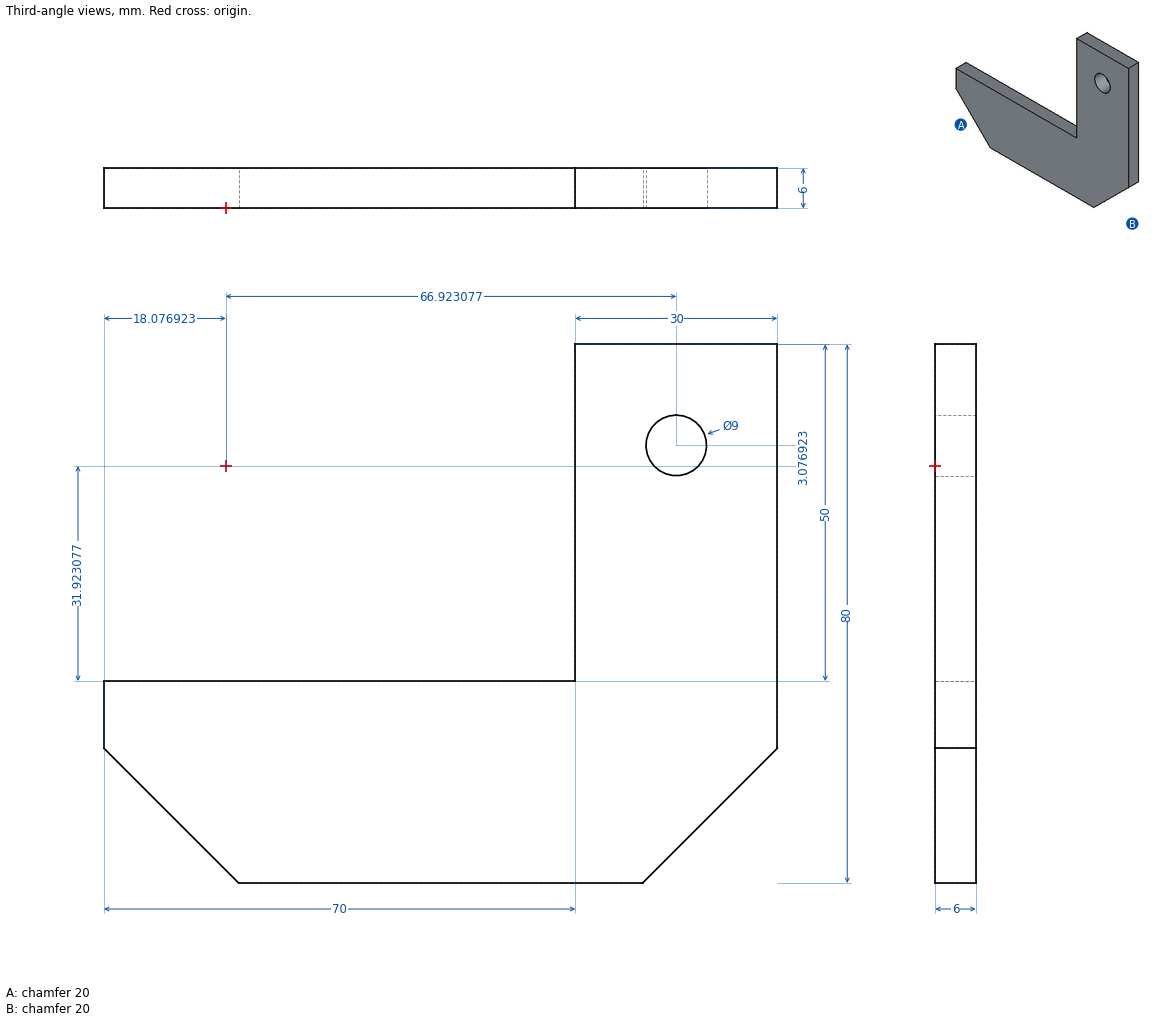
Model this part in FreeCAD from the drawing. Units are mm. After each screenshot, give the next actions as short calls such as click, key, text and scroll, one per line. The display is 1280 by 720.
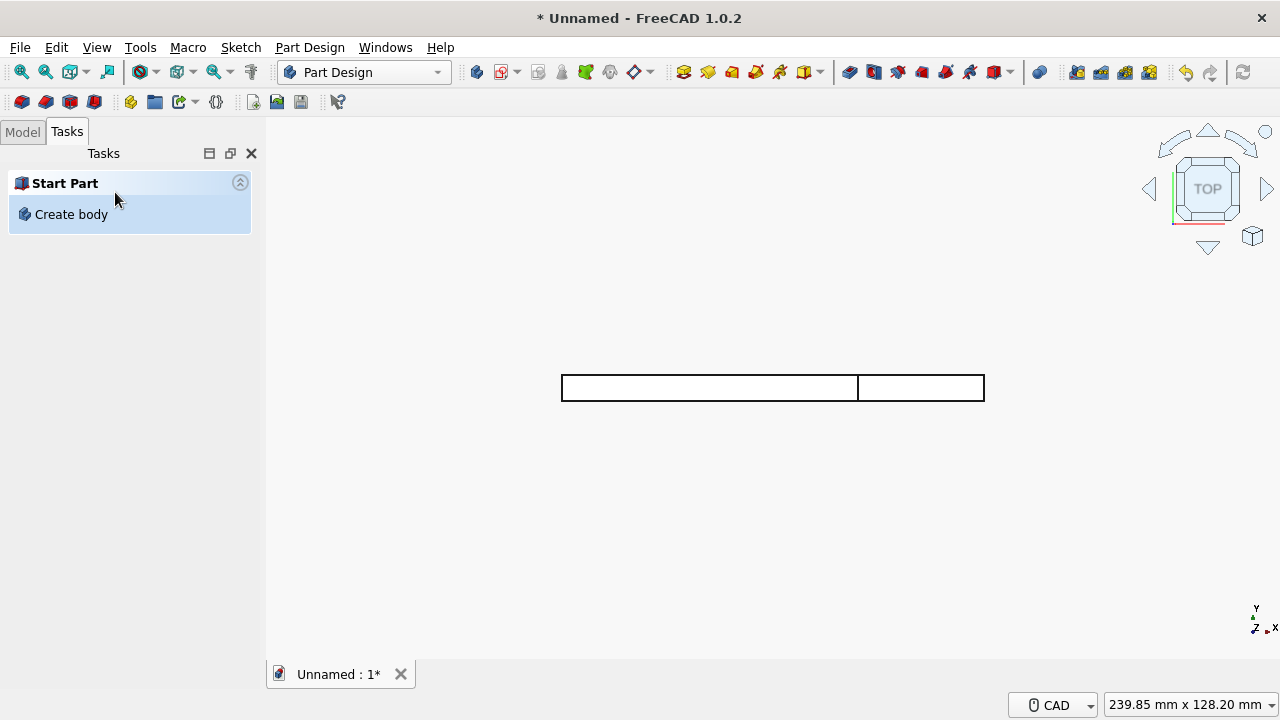
click(22, 72)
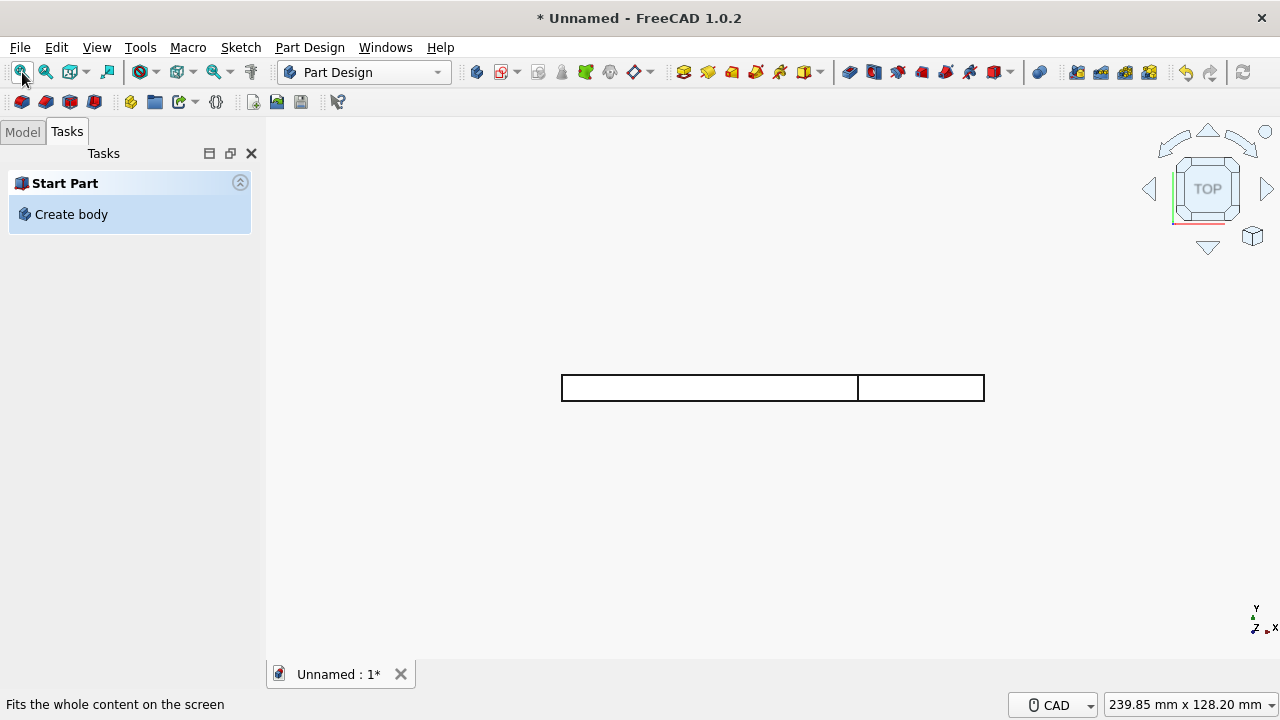
key(1)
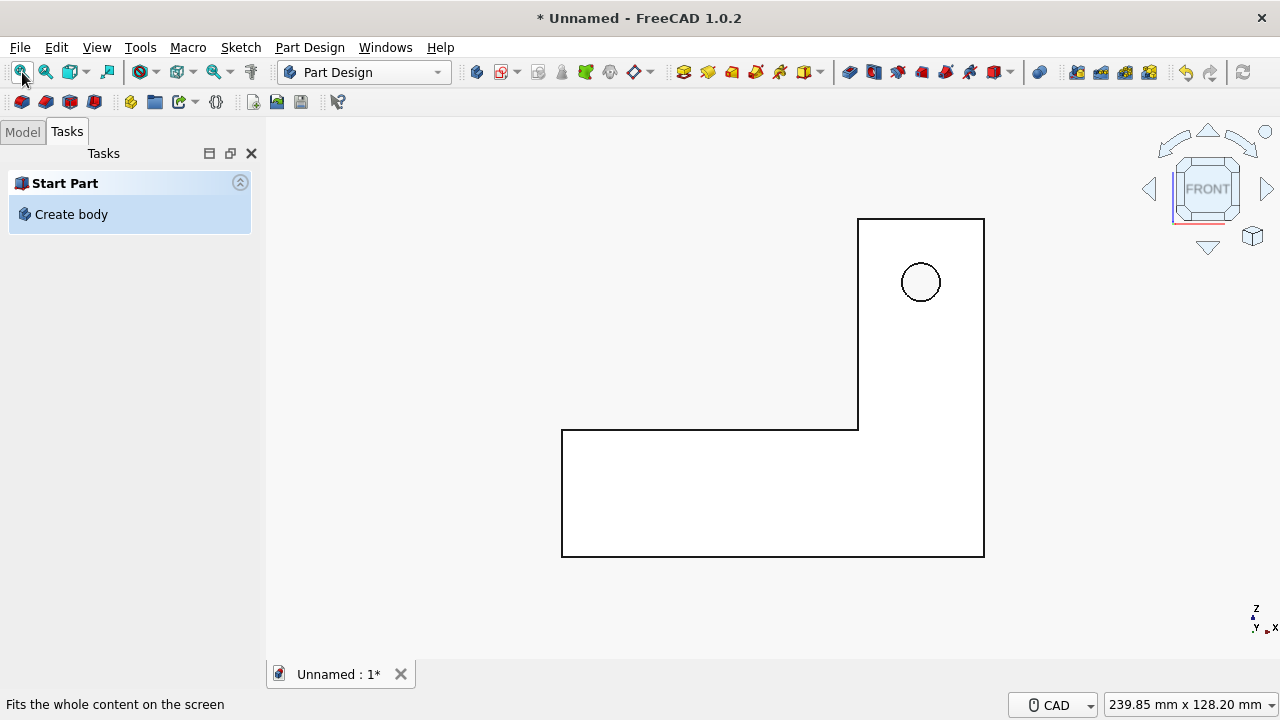
key(3)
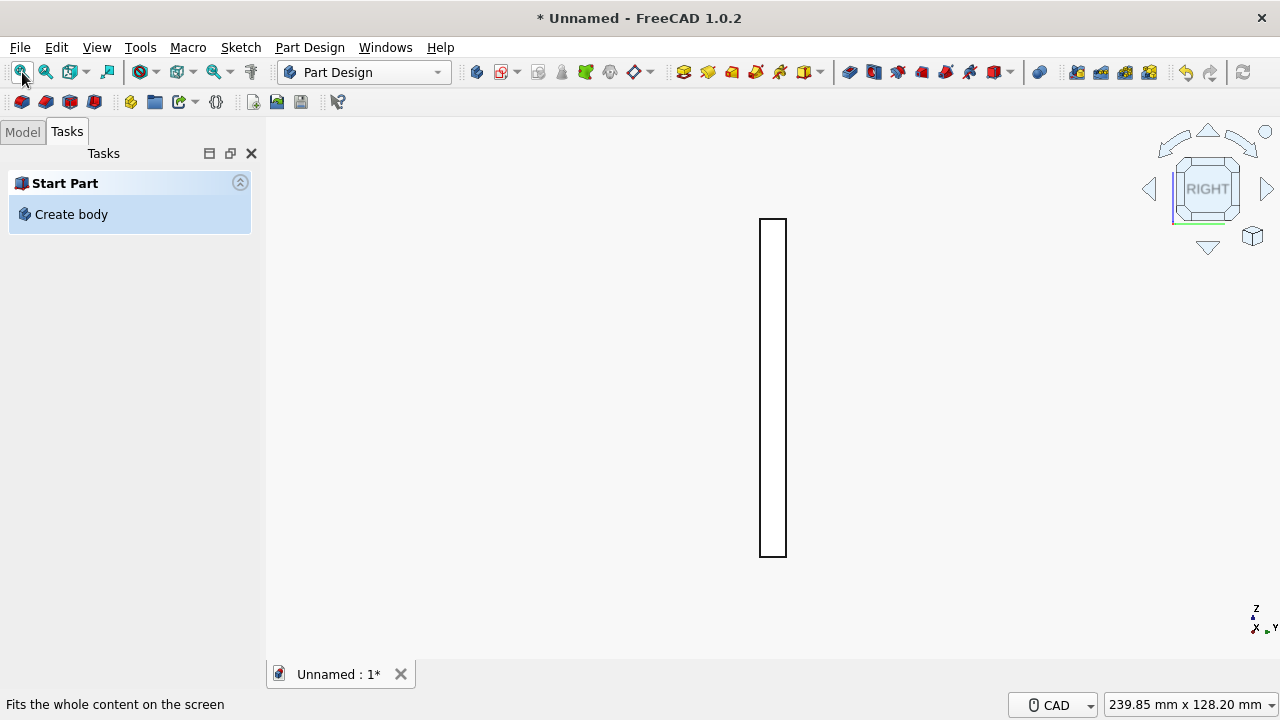
key(5)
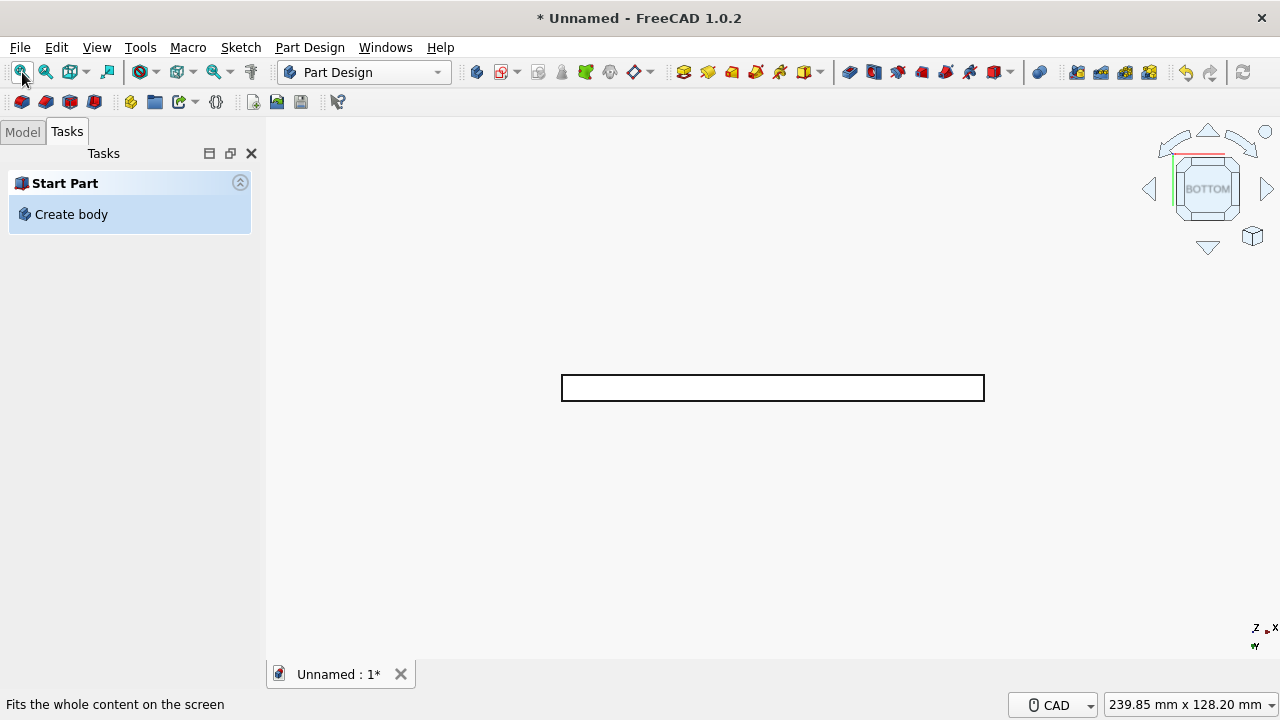
click(22, 72)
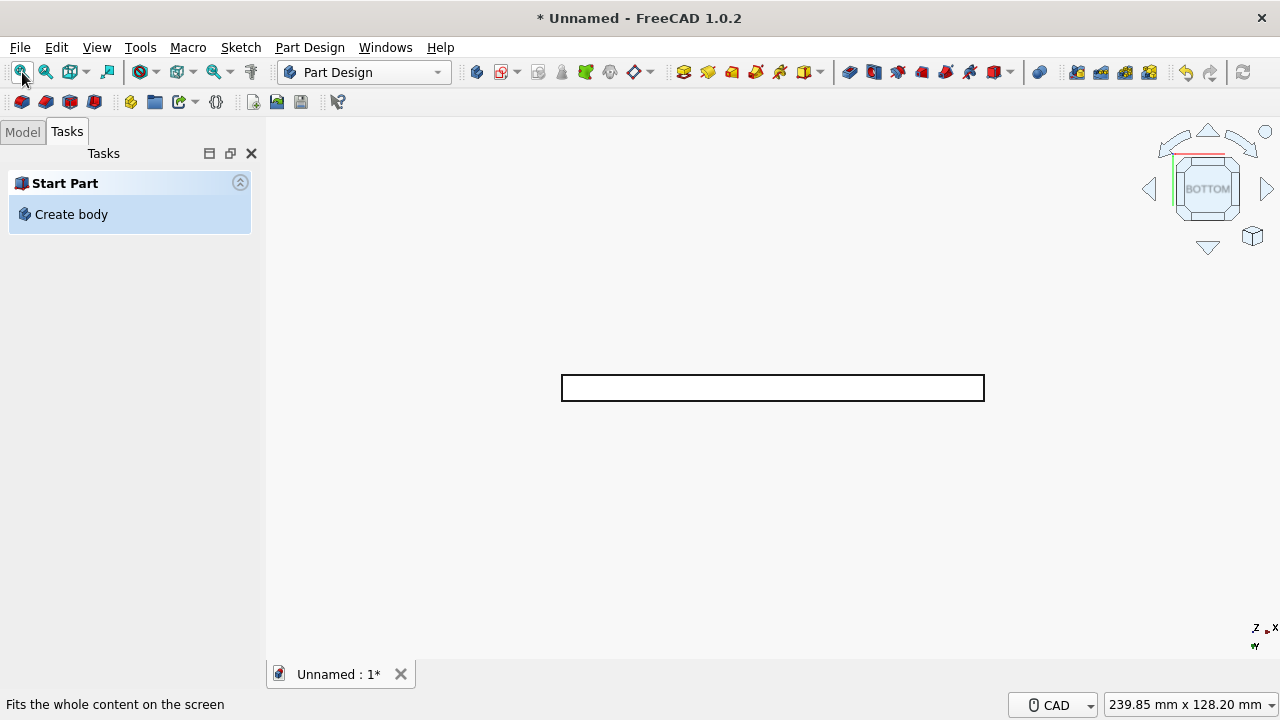
click(562, 387)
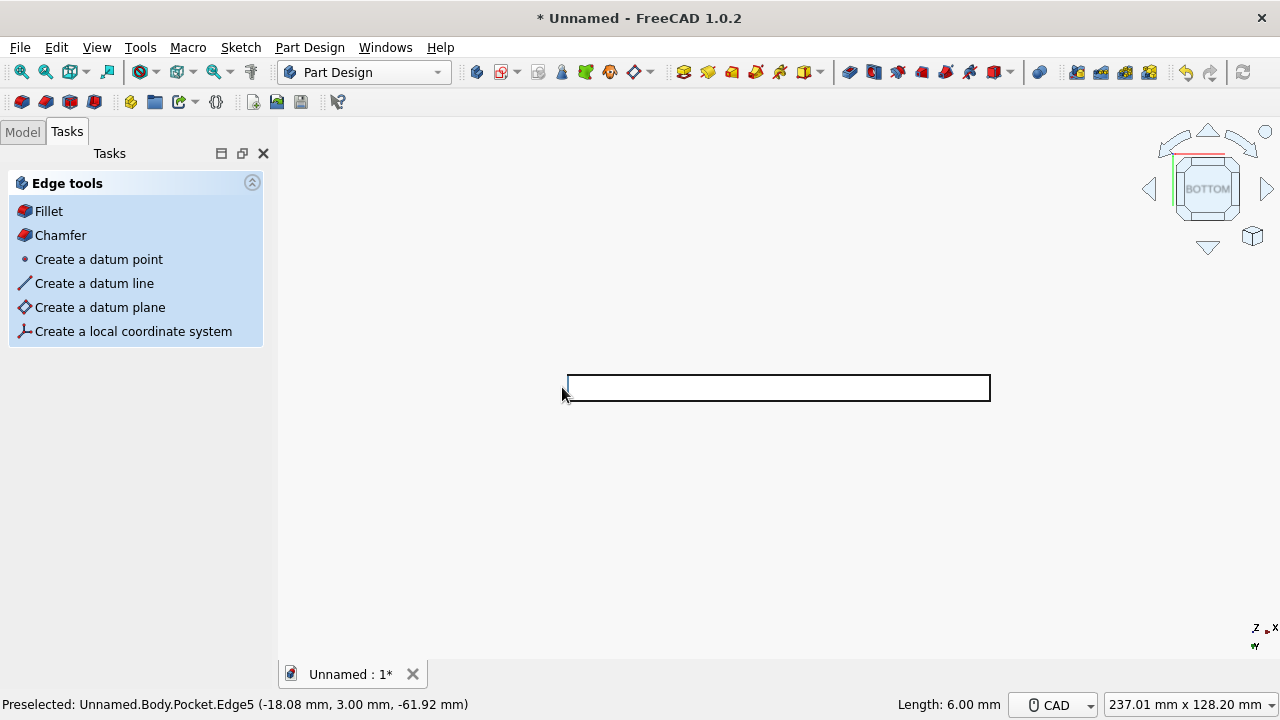
click(46, 102)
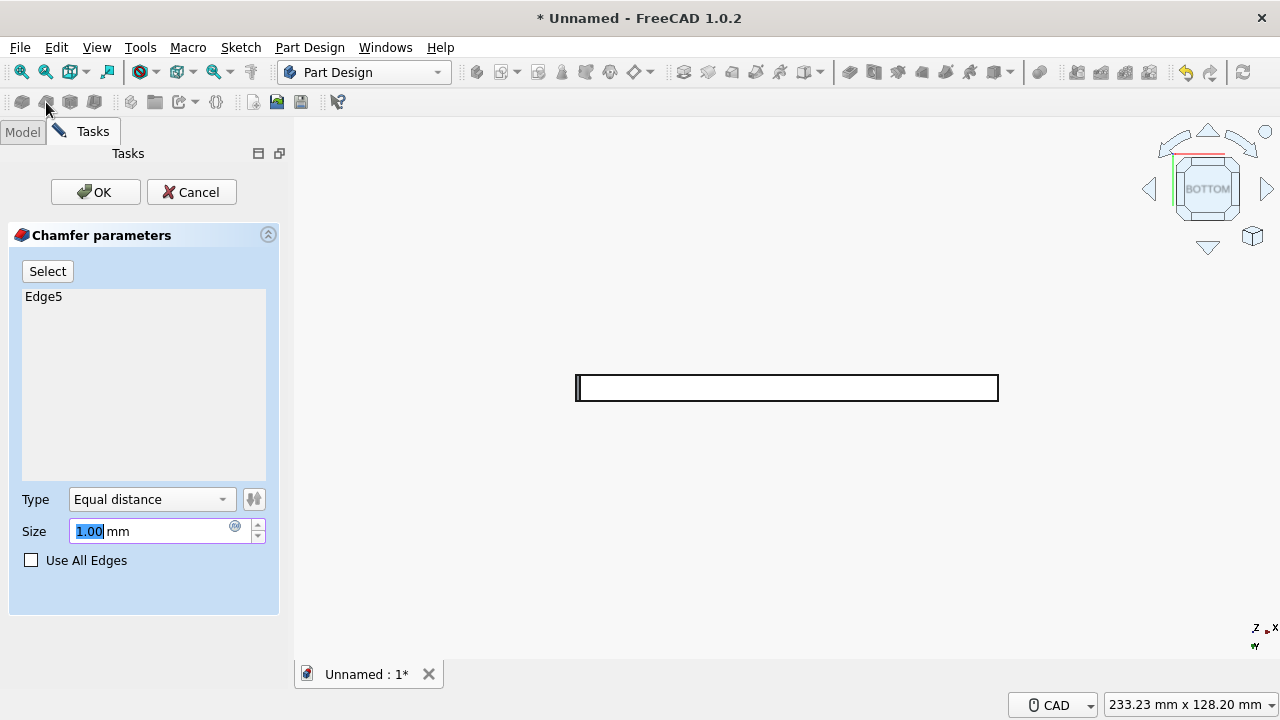
text(20)
key(Tab)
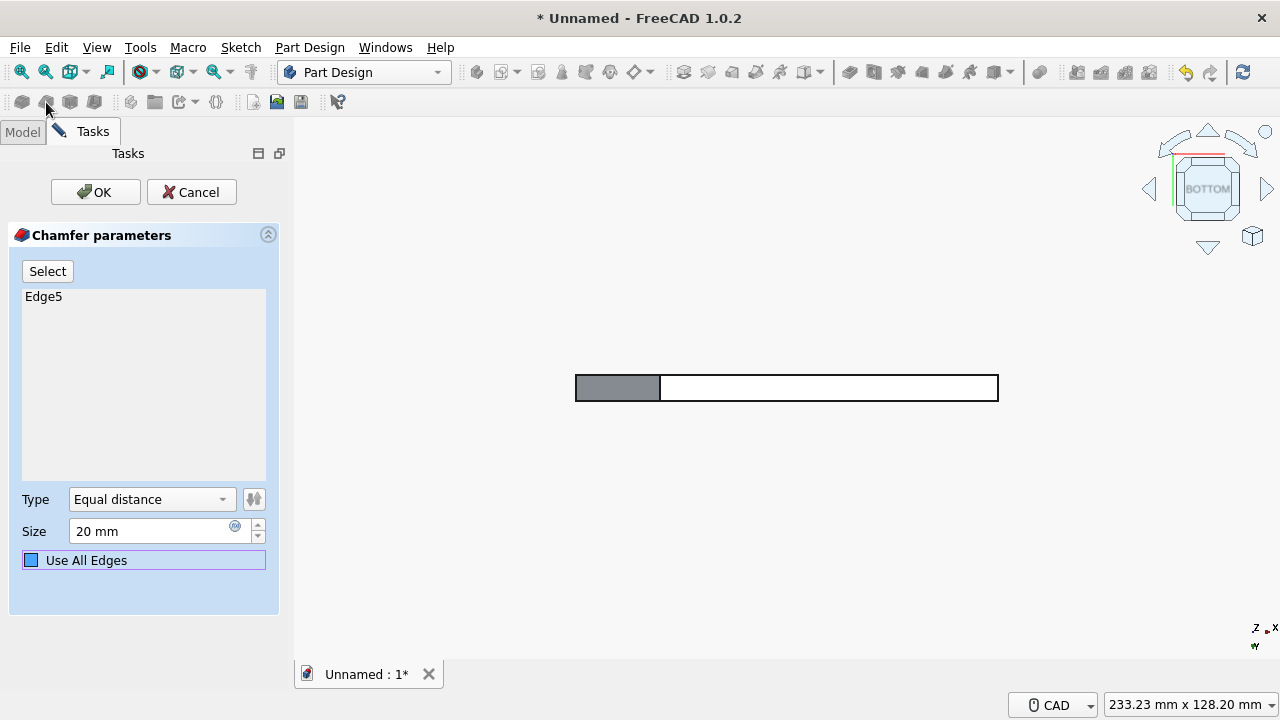
click(96, 192)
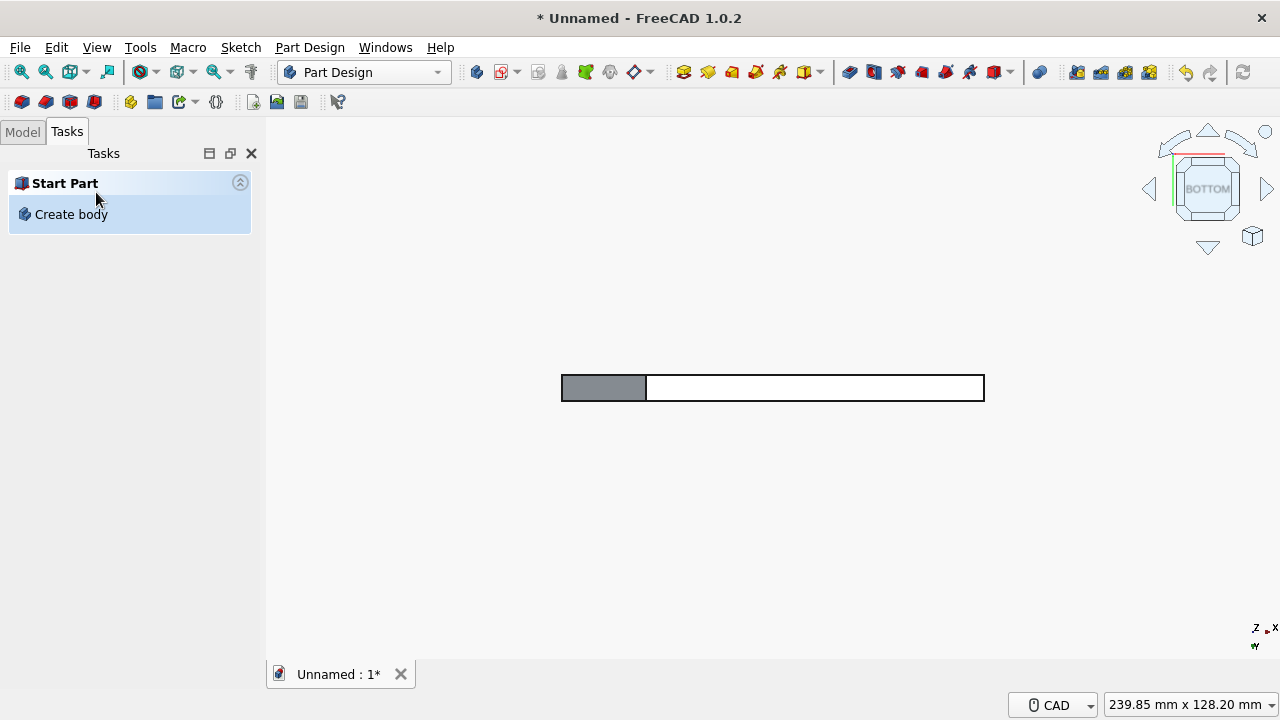
key(v)
key(f)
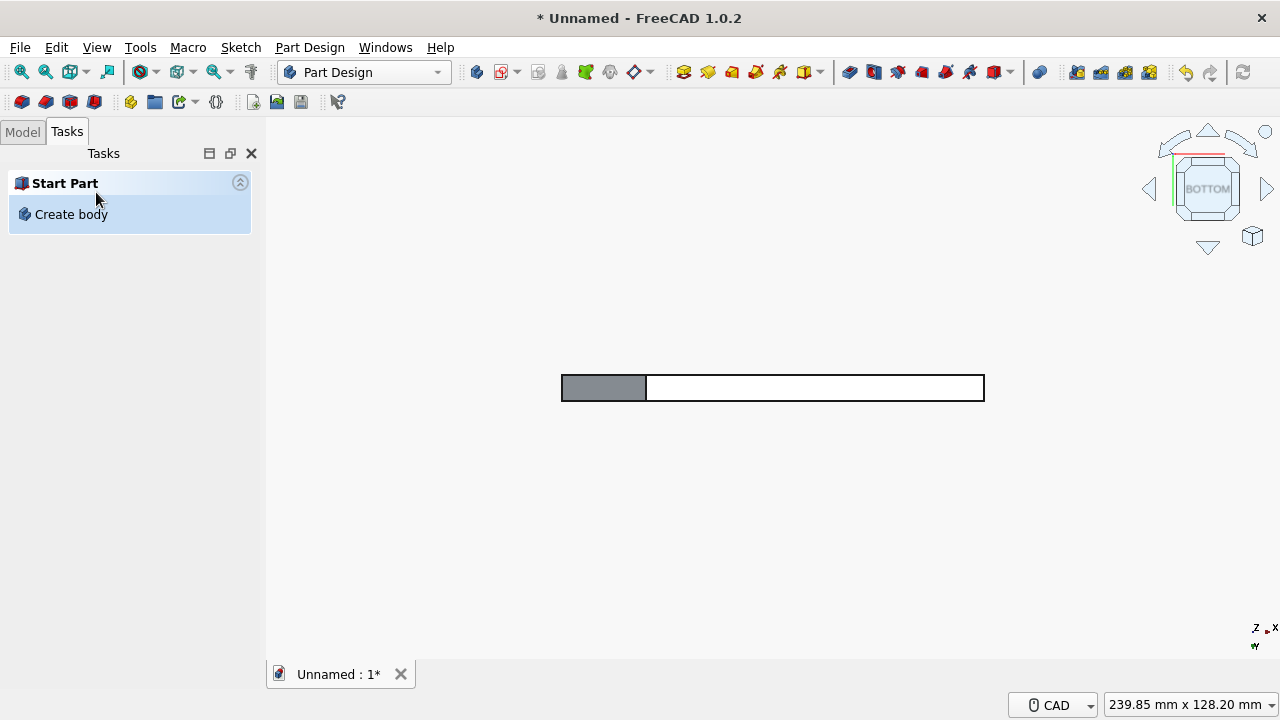
click(984, 387)